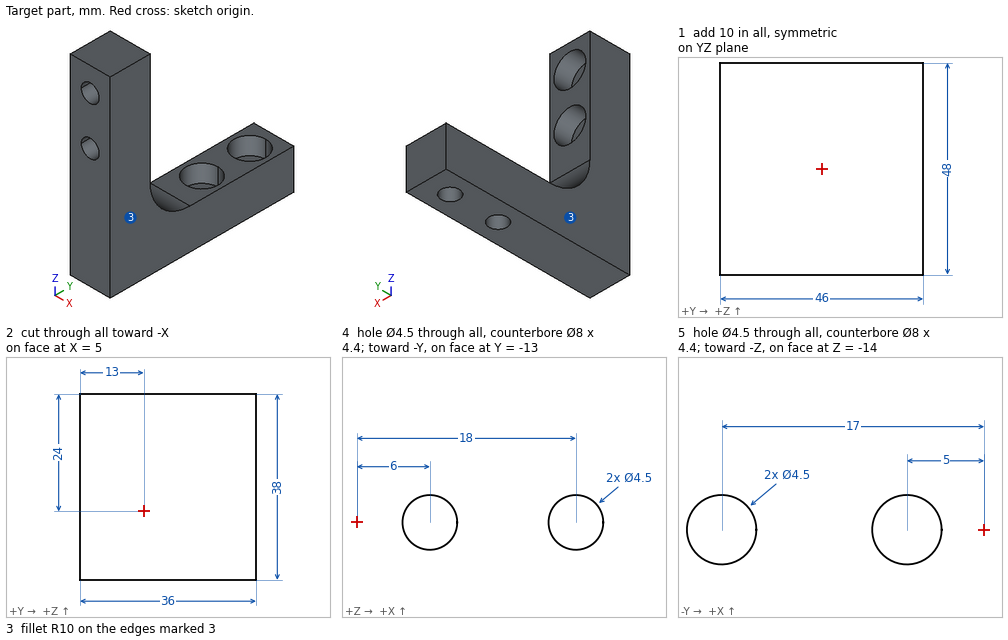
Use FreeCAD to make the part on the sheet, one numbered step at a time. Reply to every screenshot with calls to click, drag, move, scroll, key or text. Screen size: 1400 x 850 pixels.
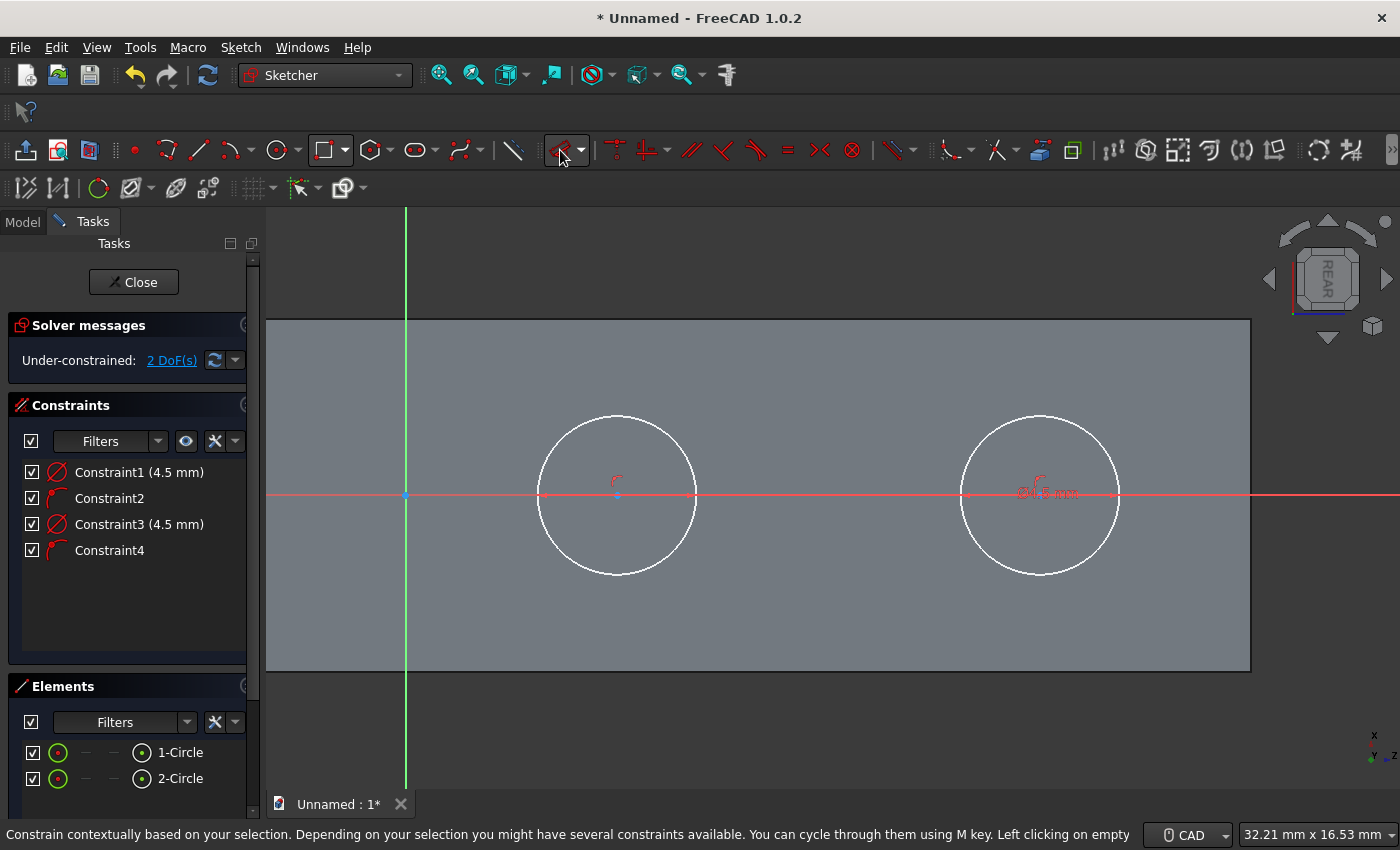
click(617, 495)
click(511, 529)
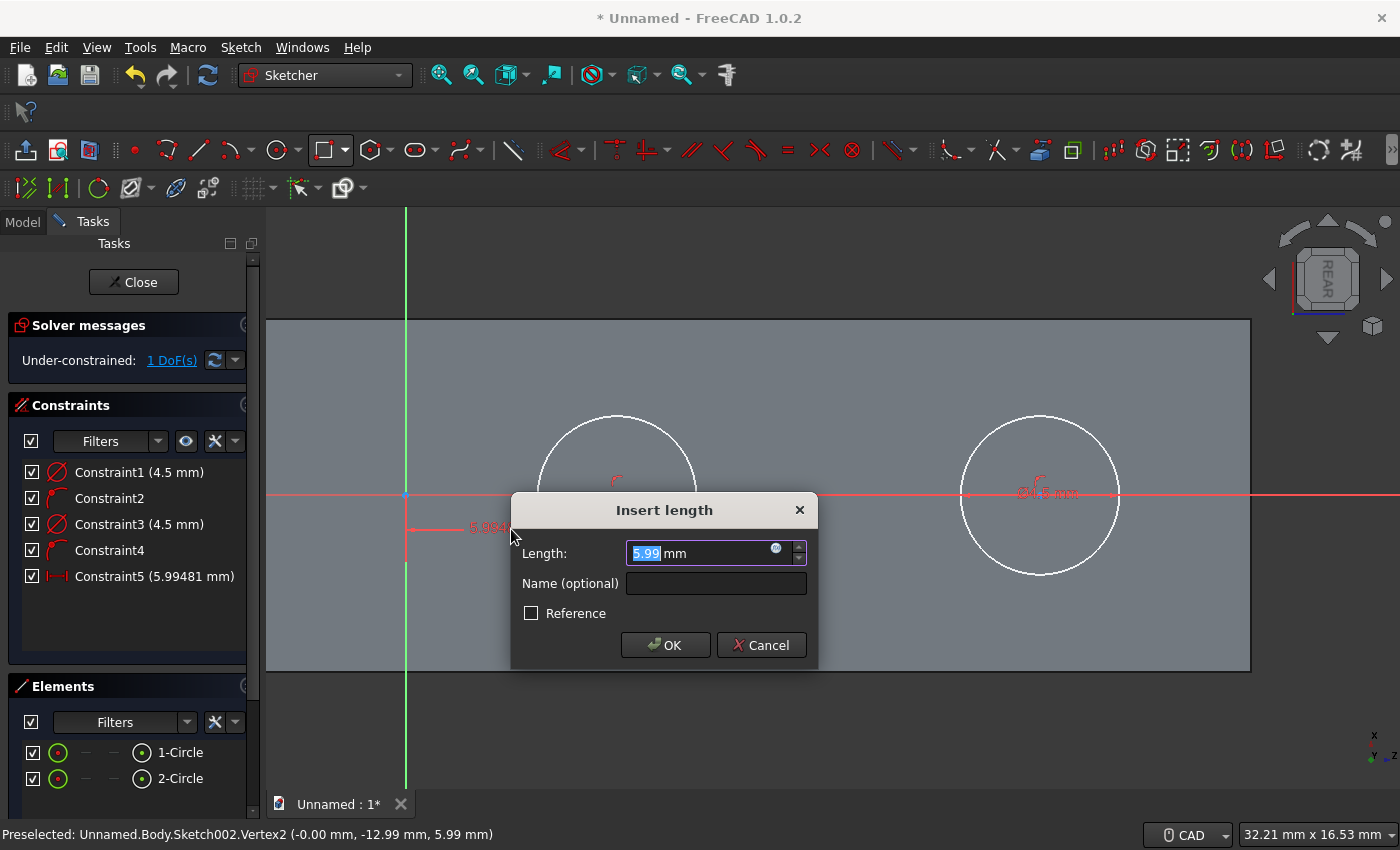
text(6)
key(Return)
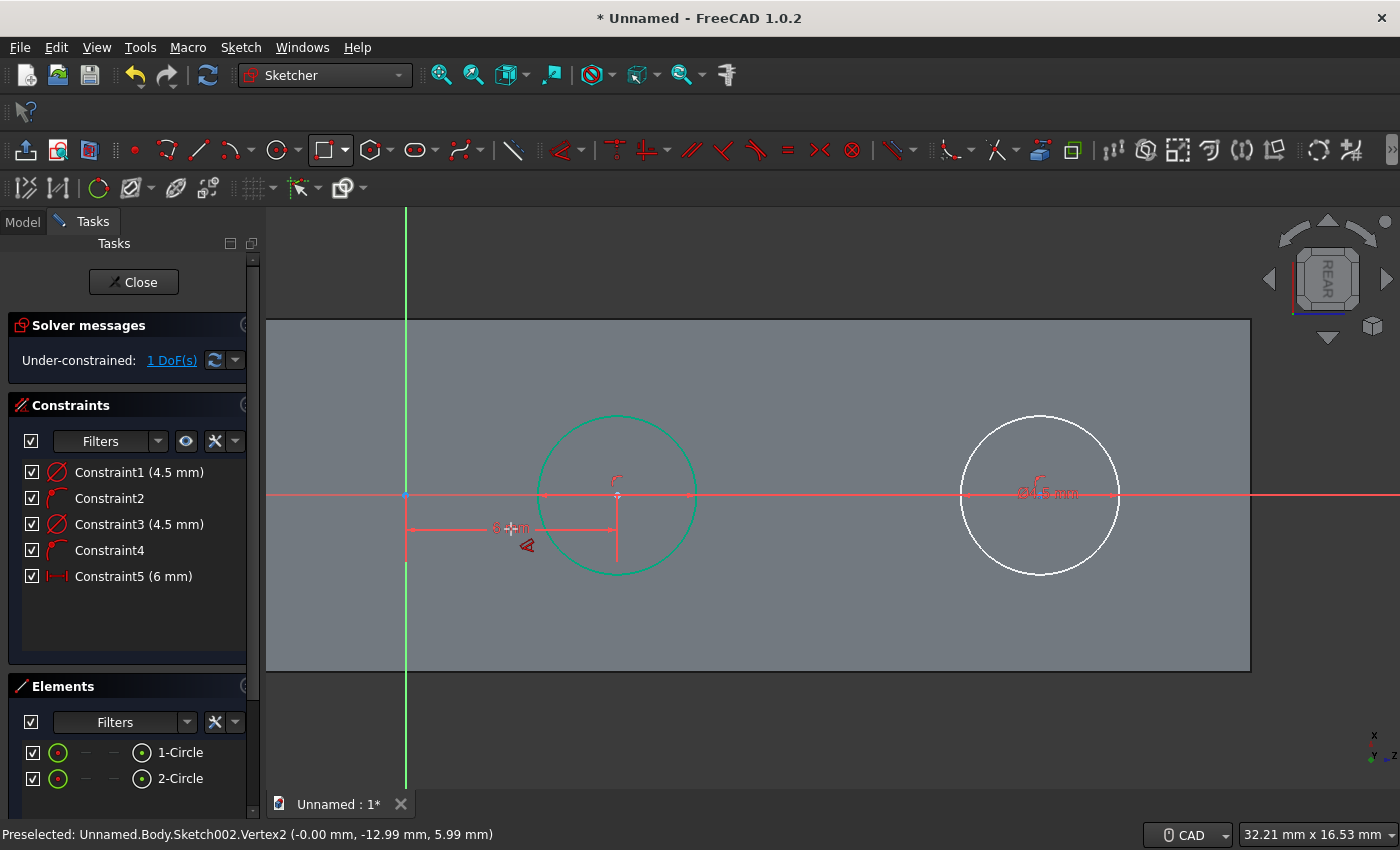
click(1040, 495)
click(723, 529)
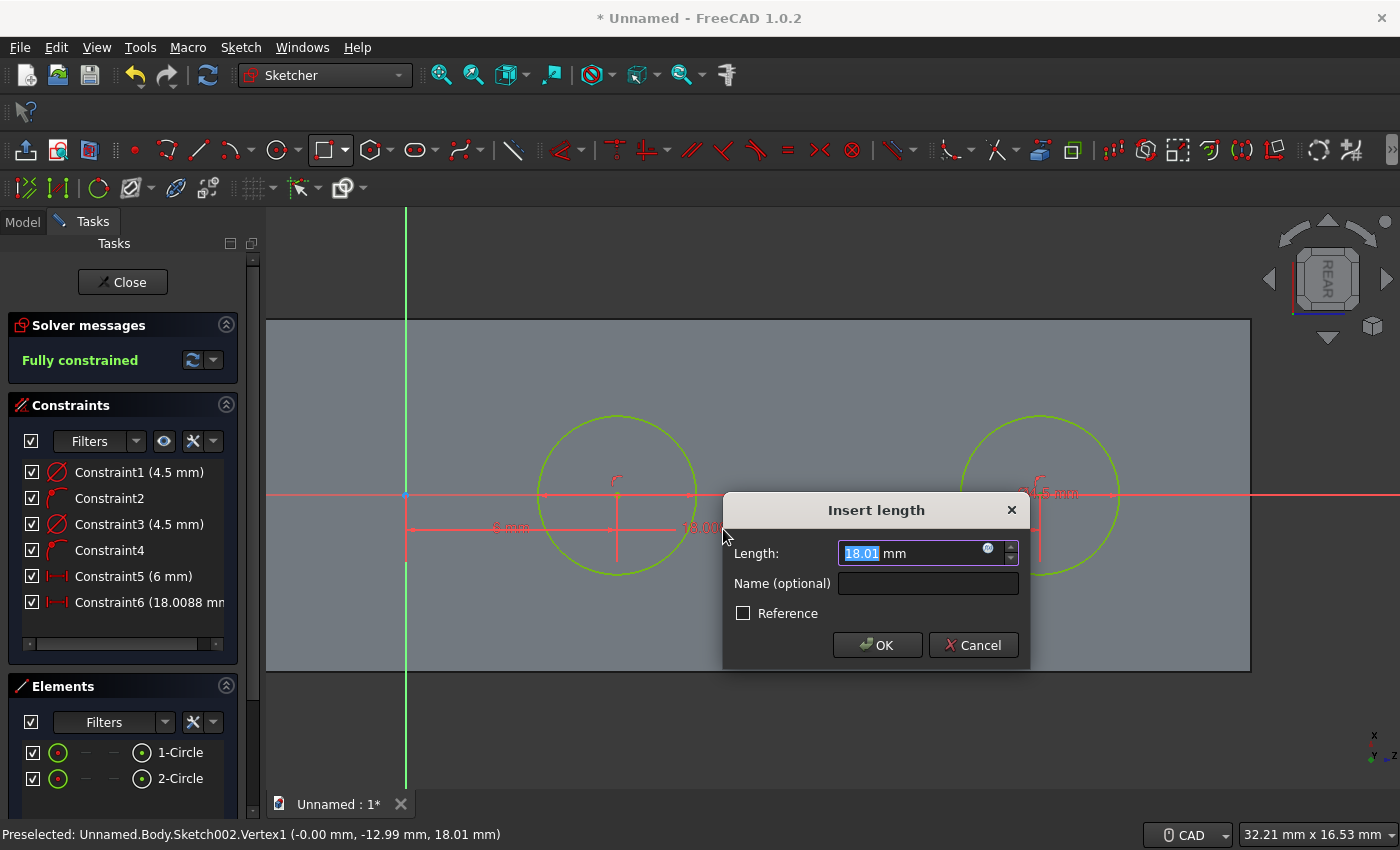
text(18)
key(Return)
key(Escape)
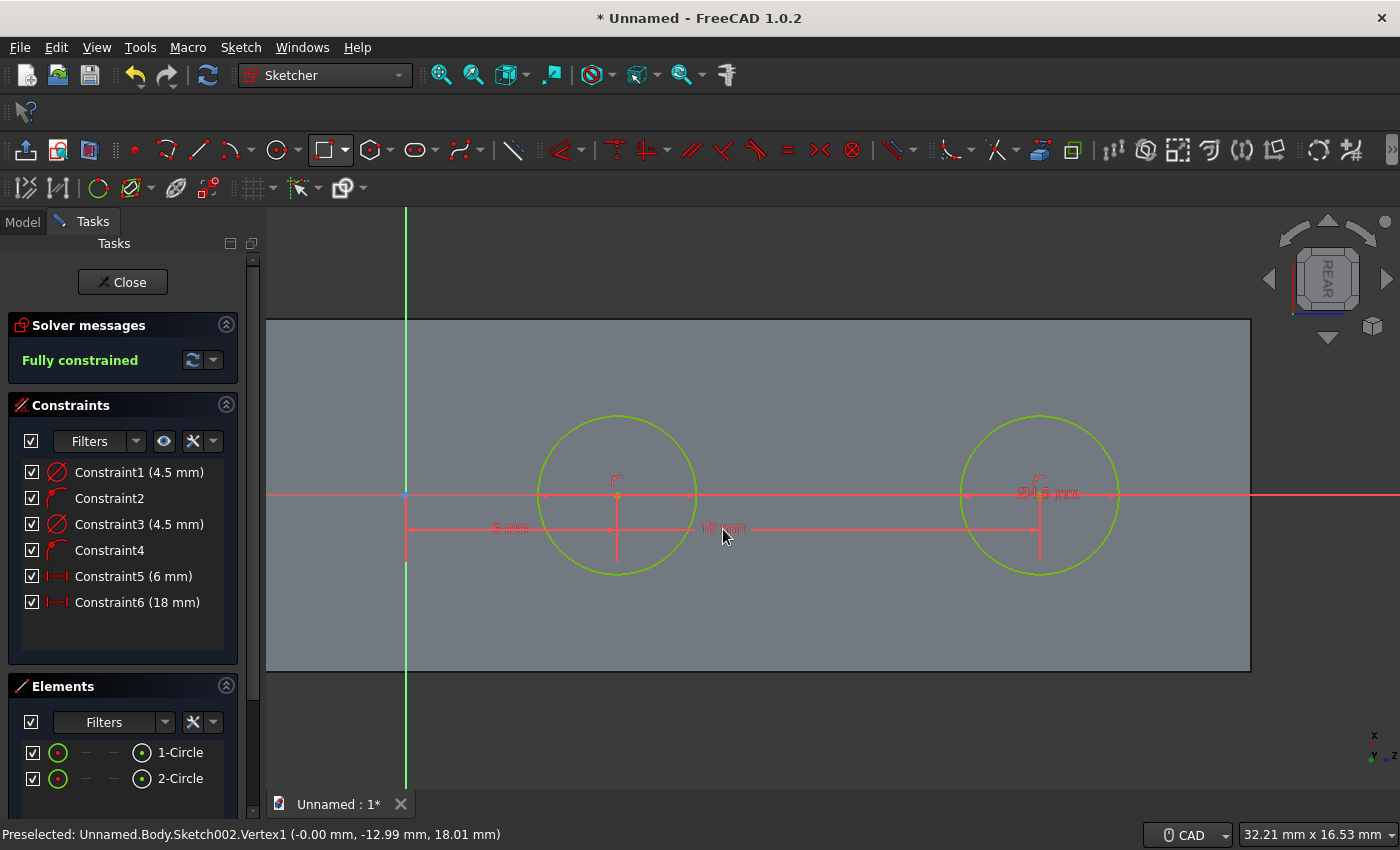
click(123, 282)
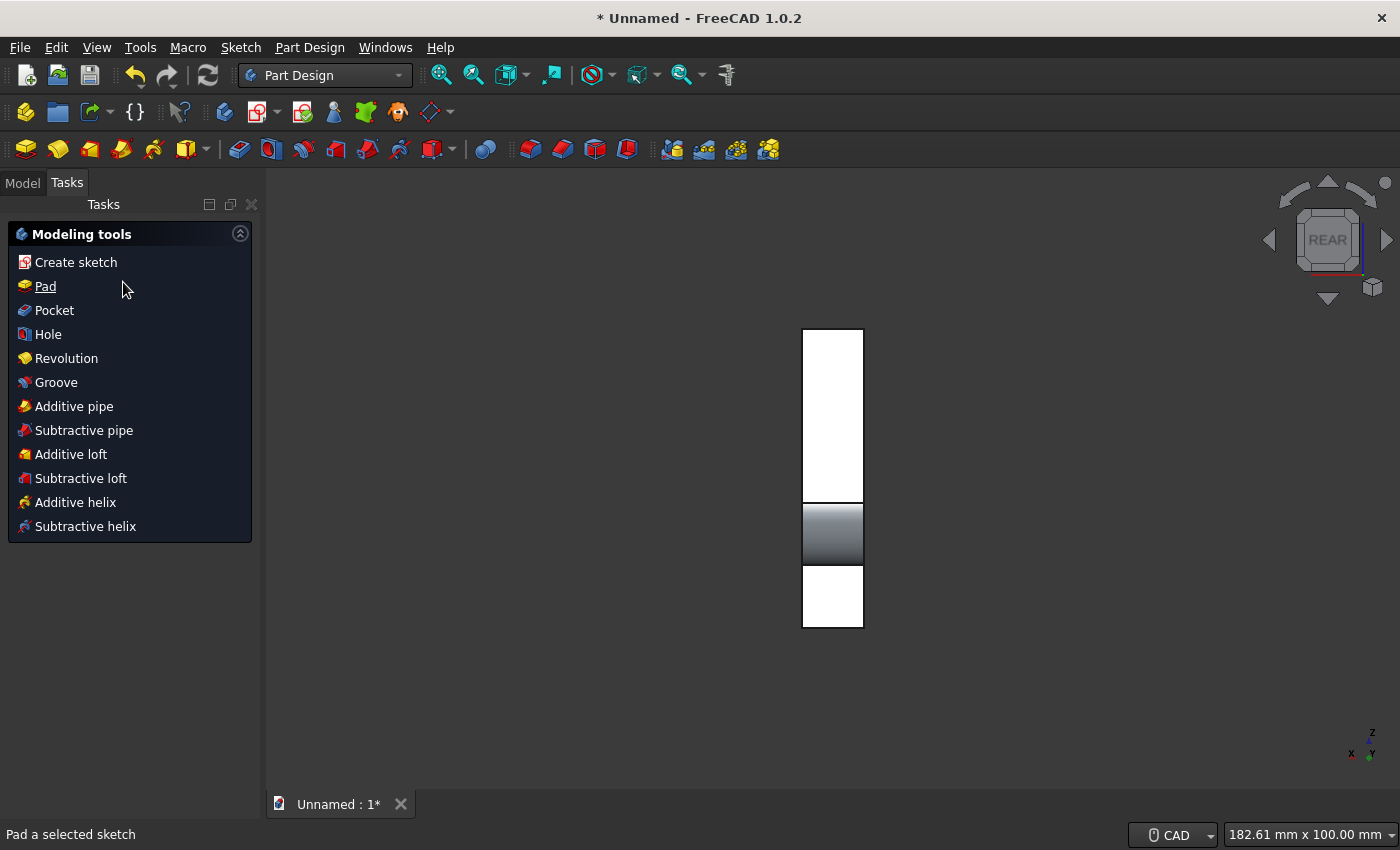
click(272, 150)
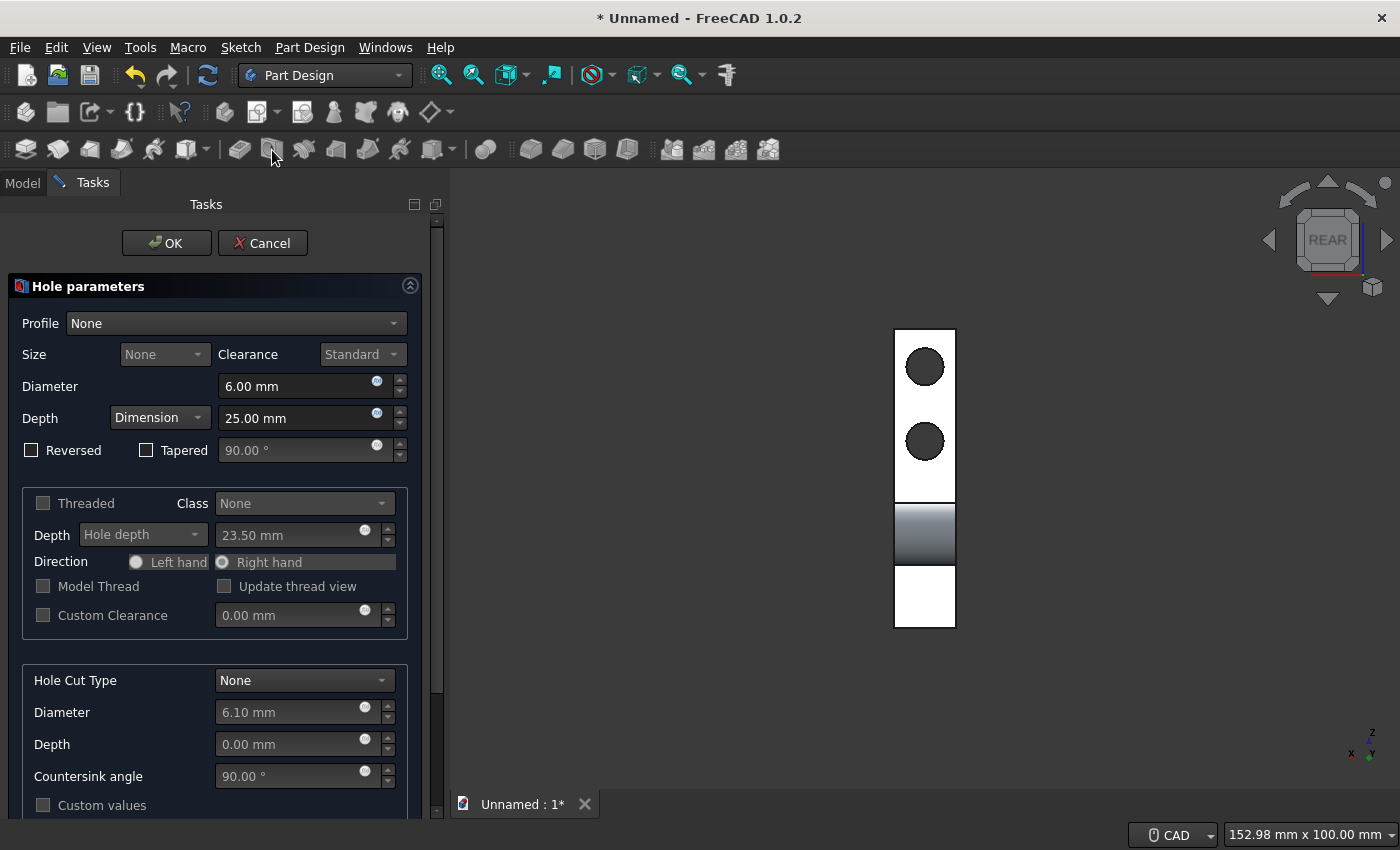
triple_click(305, 386)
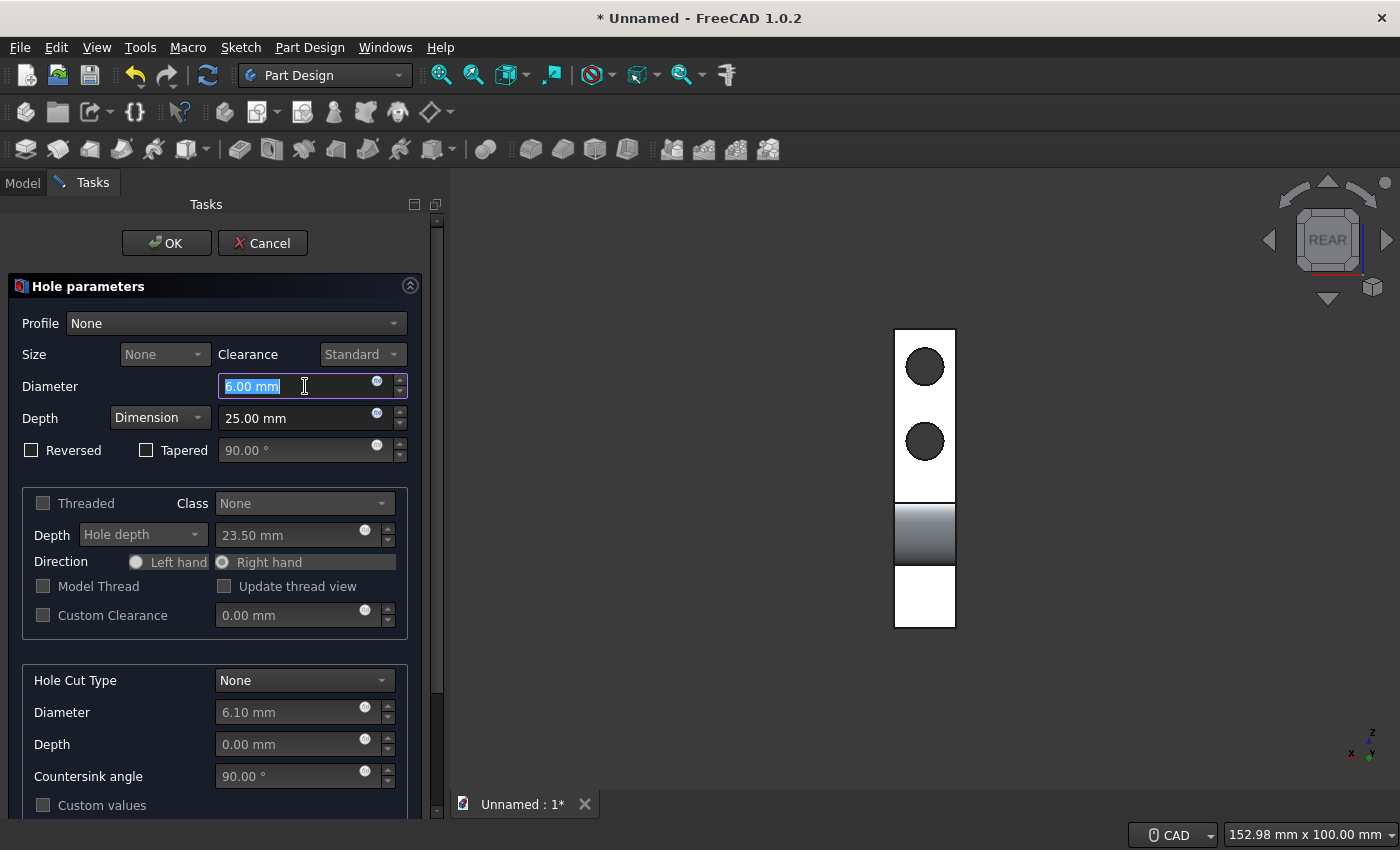
text(4.5)
key(Tab)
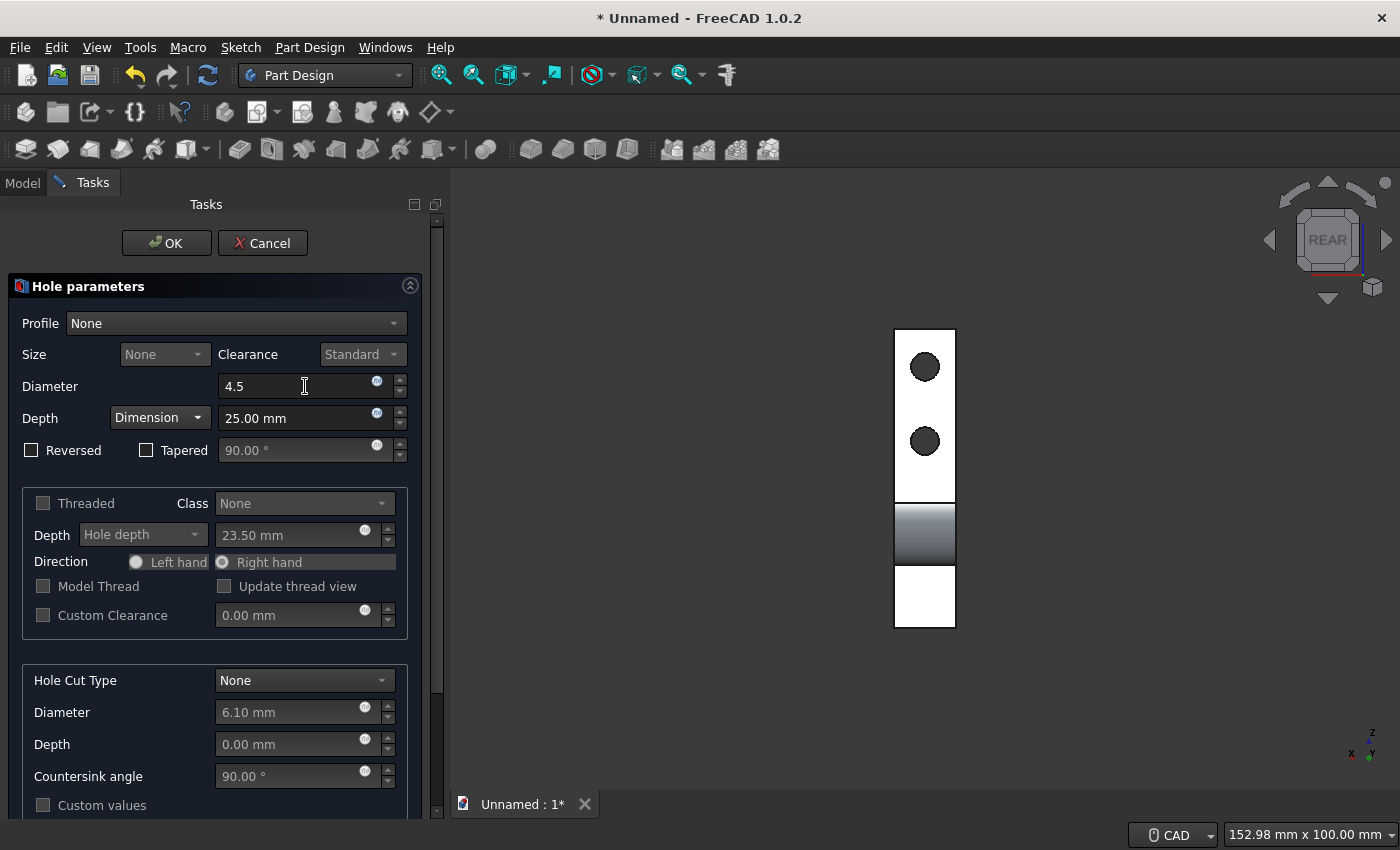
click(161, 418)